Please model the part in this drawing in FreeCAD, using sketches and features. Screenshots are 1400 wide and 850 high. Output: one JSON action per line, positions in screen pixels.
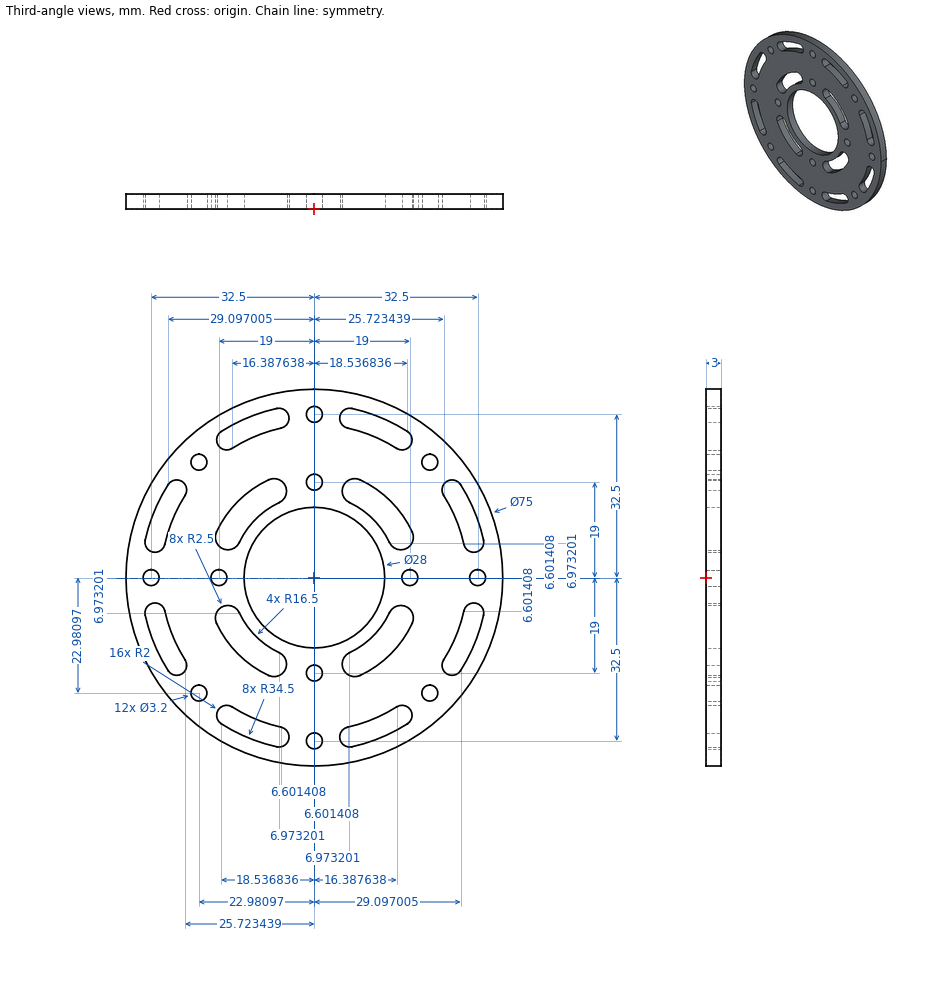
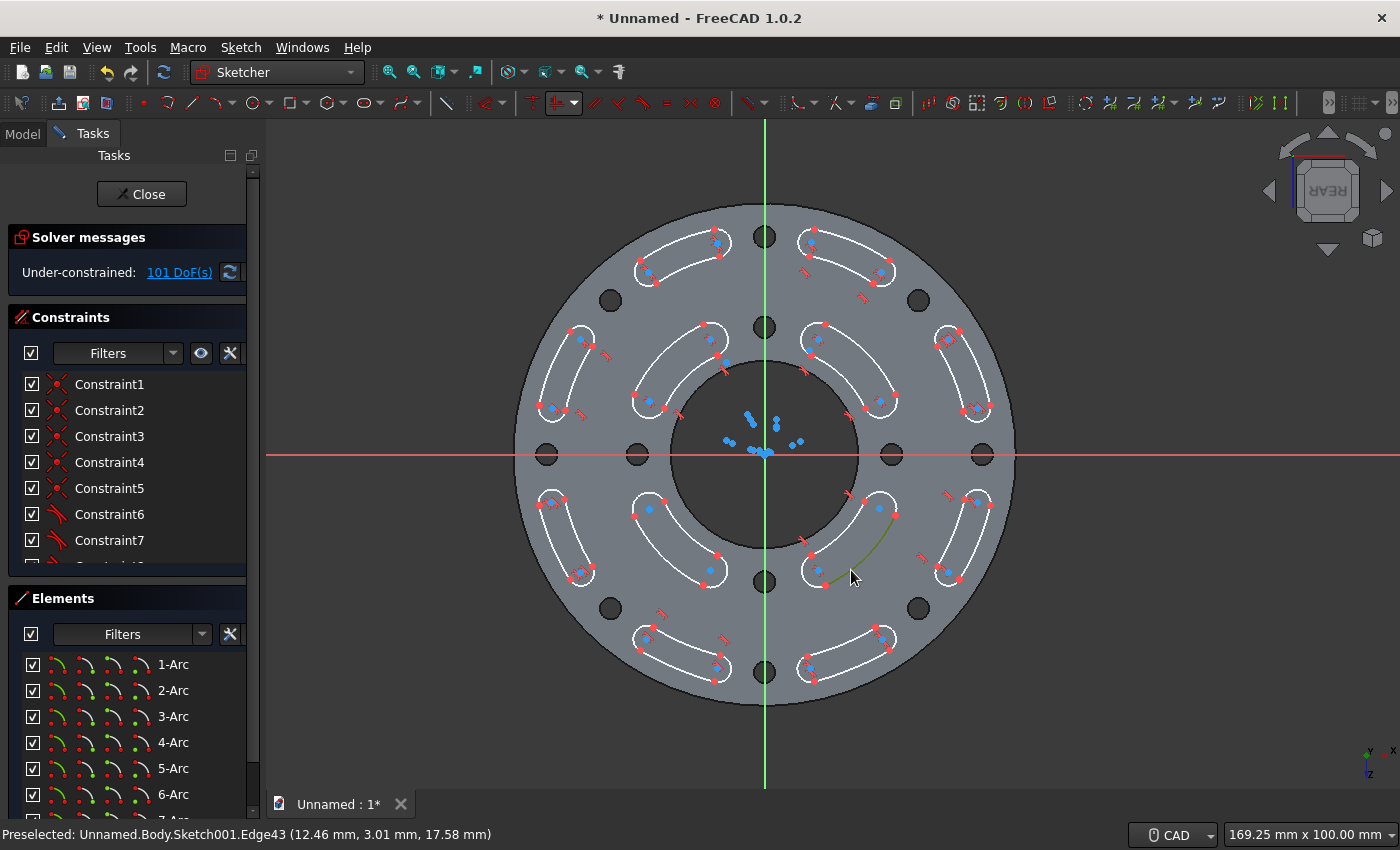
{"action": "left_click", "coordinate": [894, 501]}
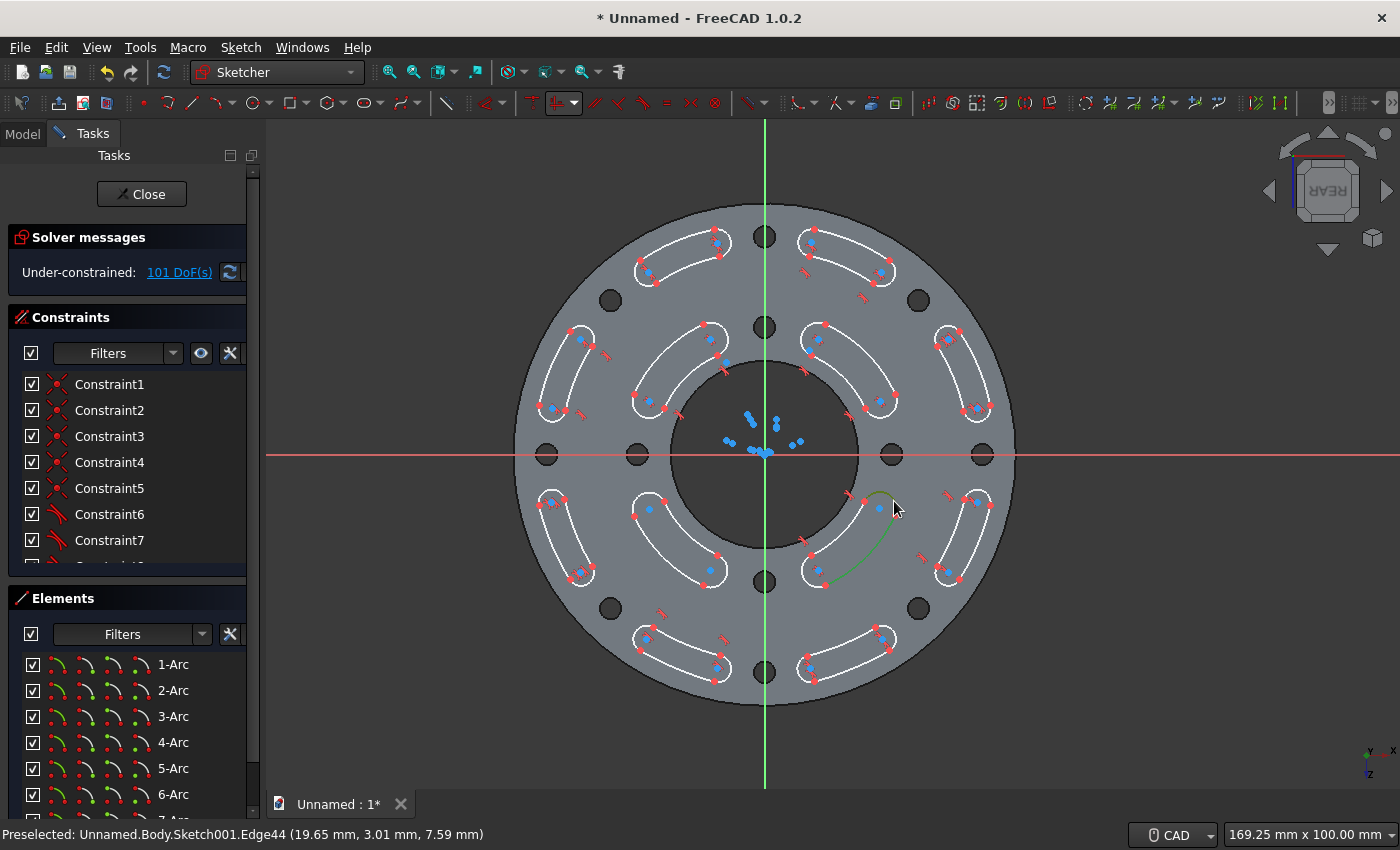
{"action": "left_click", "coordinate": [644, 104]}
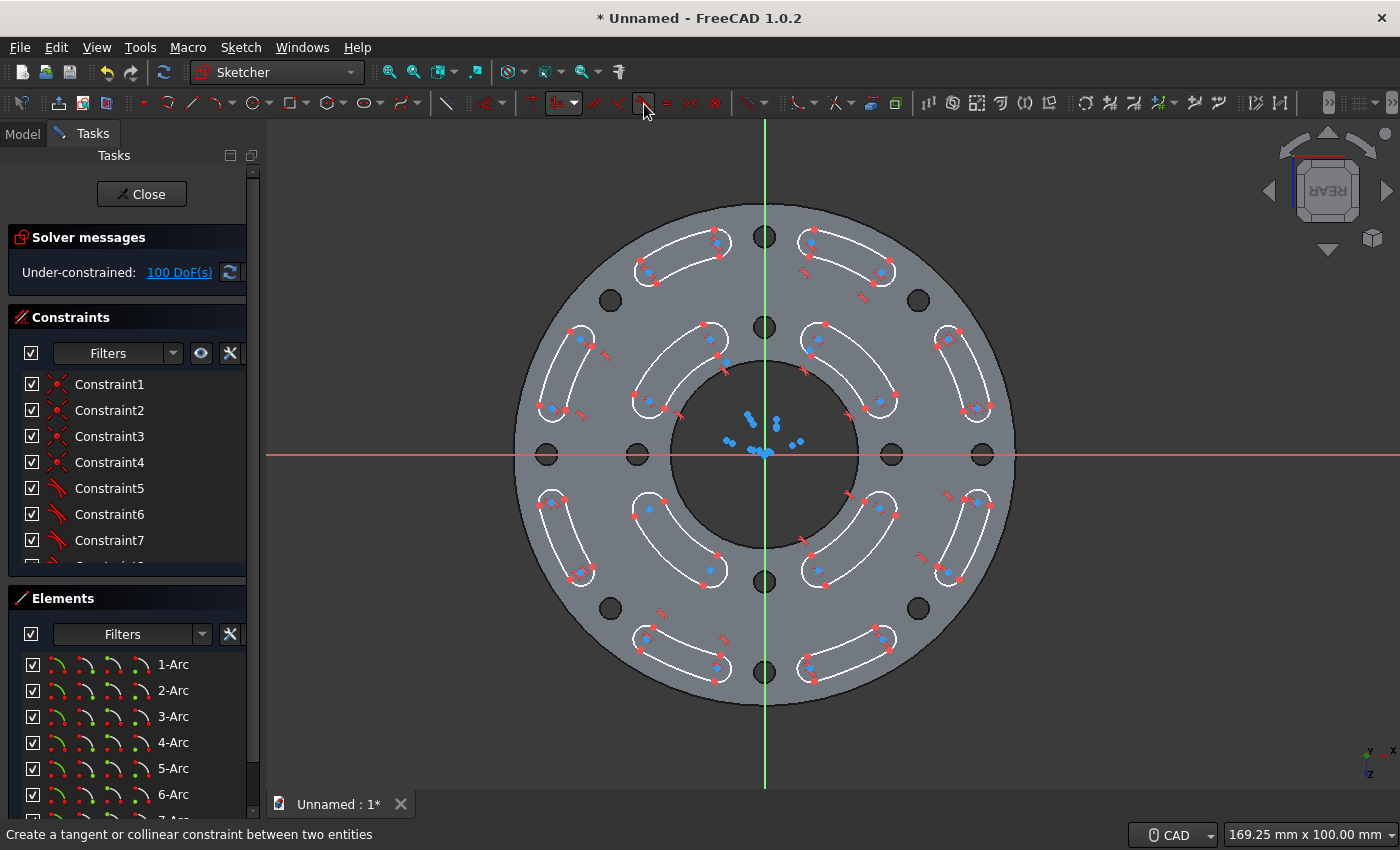
{"action": "left_click", "coordinate": [676, 521]}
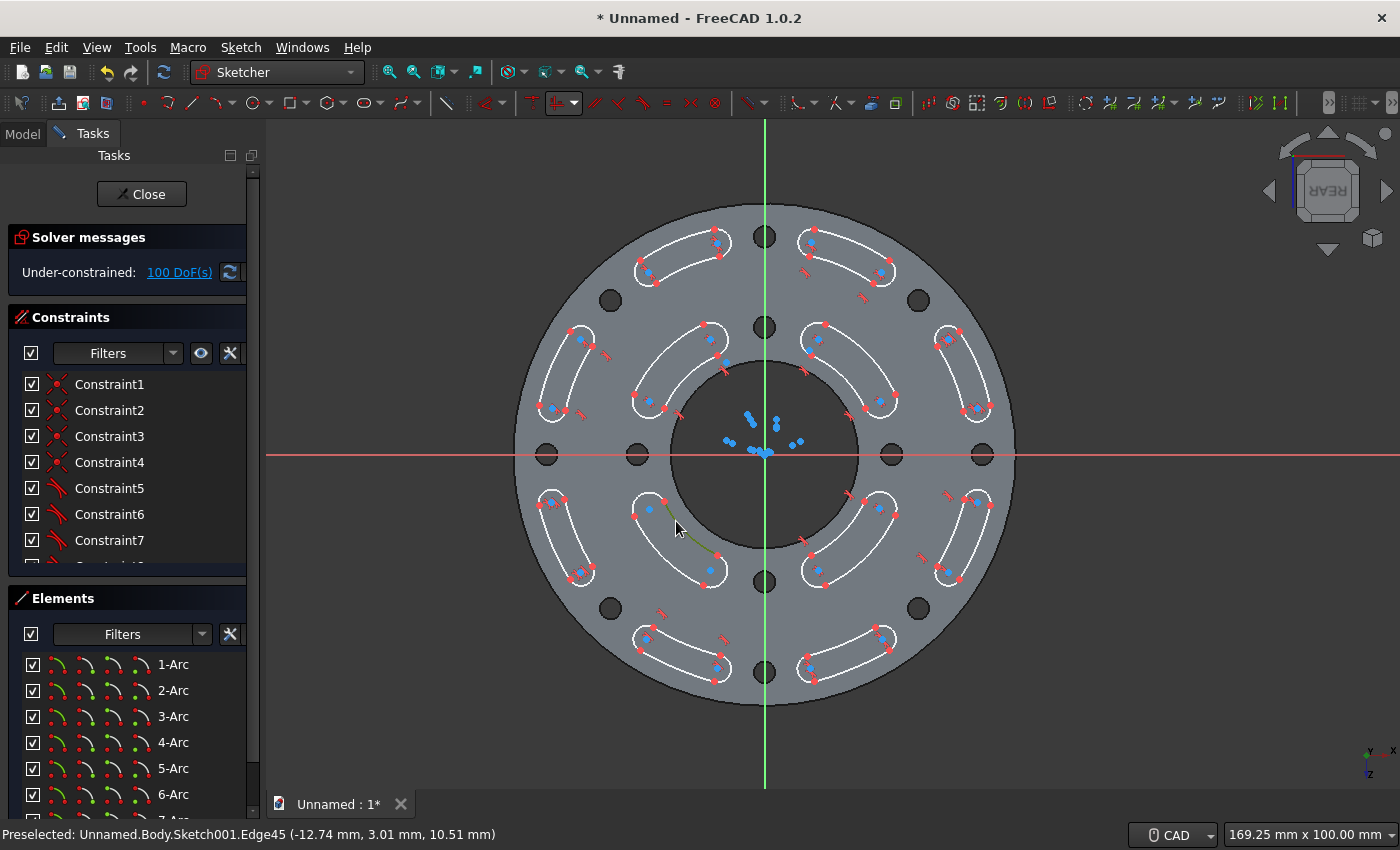
{"action": "left_click", "coordinate": [652, 493]}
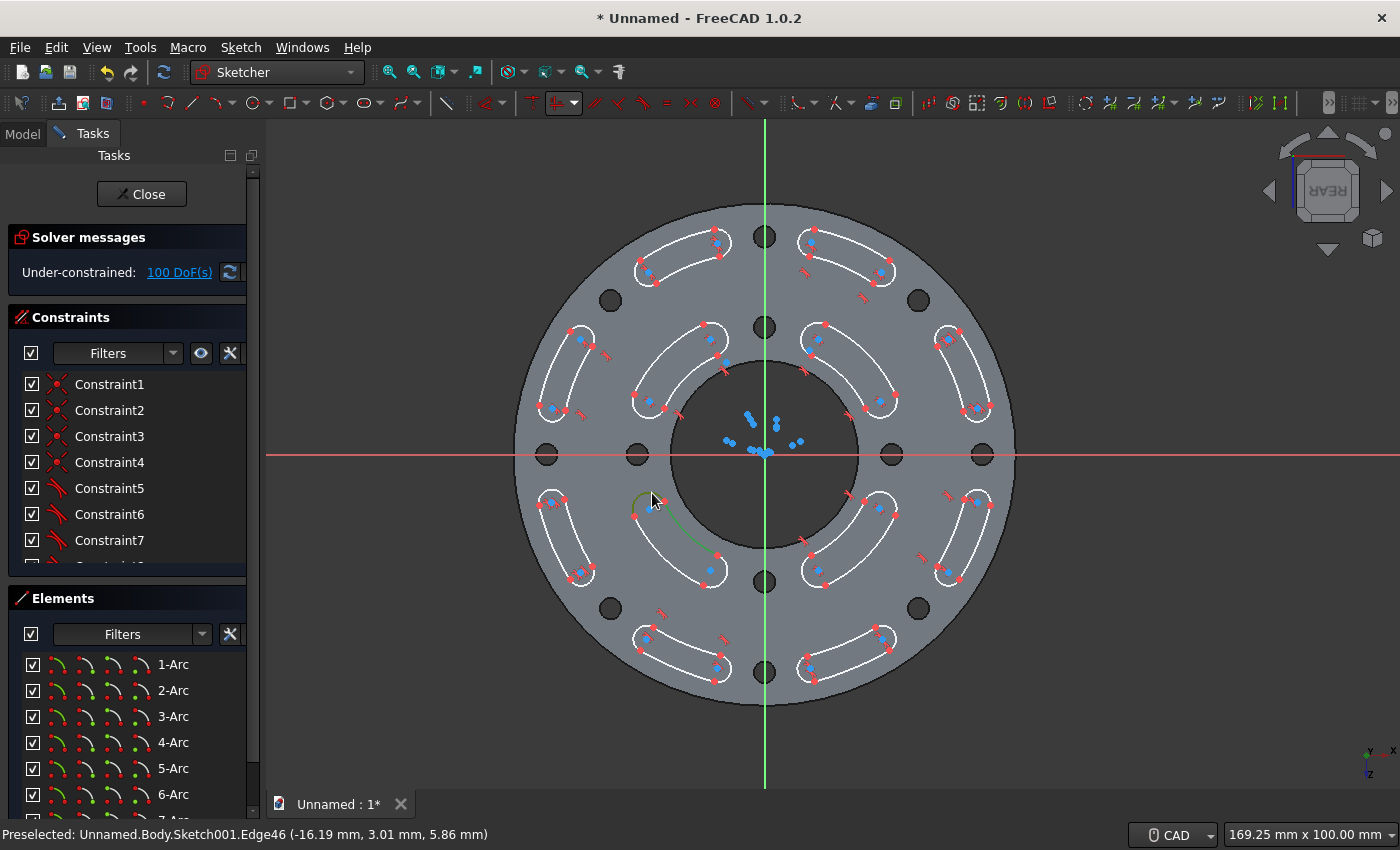
{"action": "left_click", "coordinate": [644, 104]}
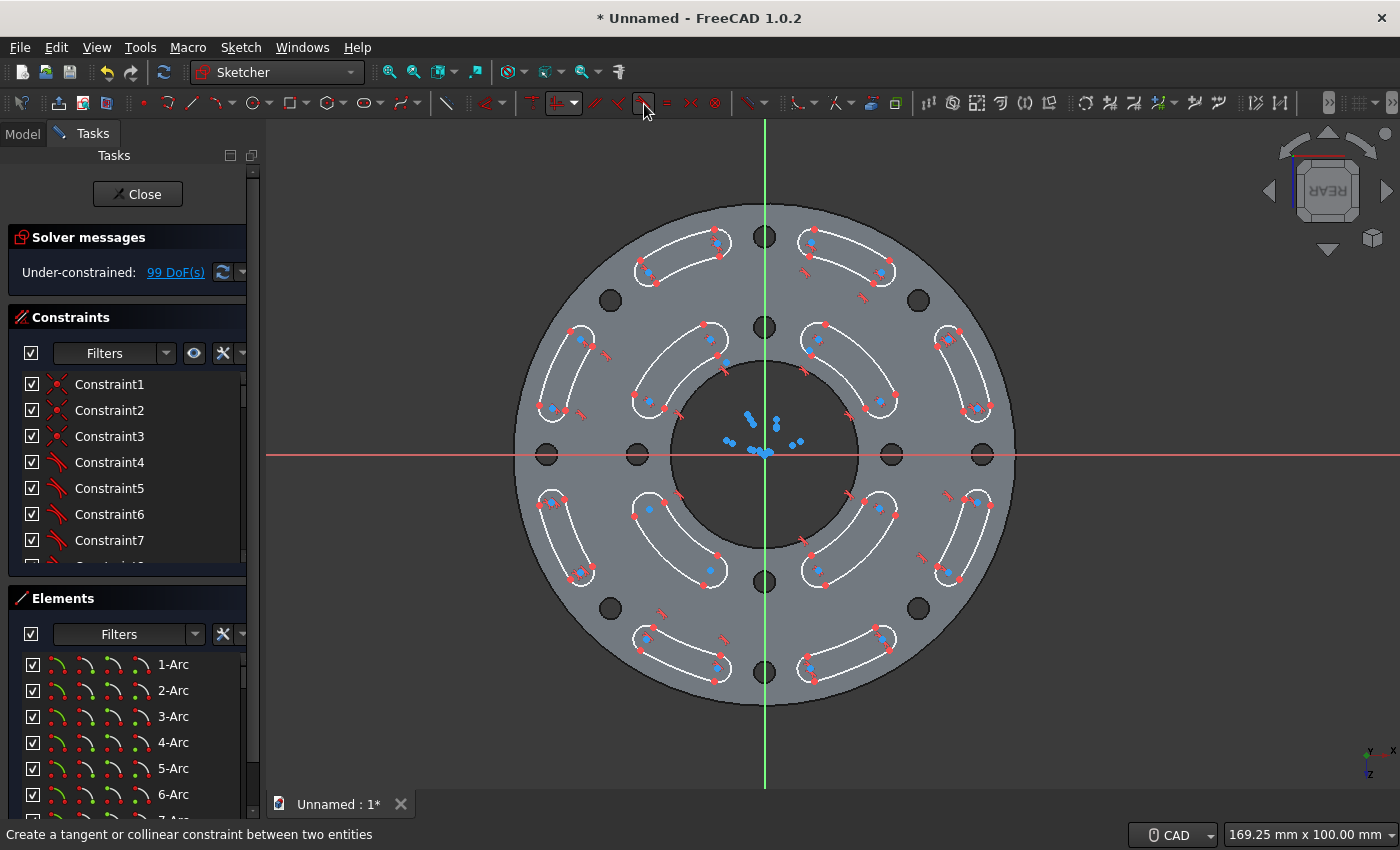
{"action": "left_click", "coordinate": [676, 522]}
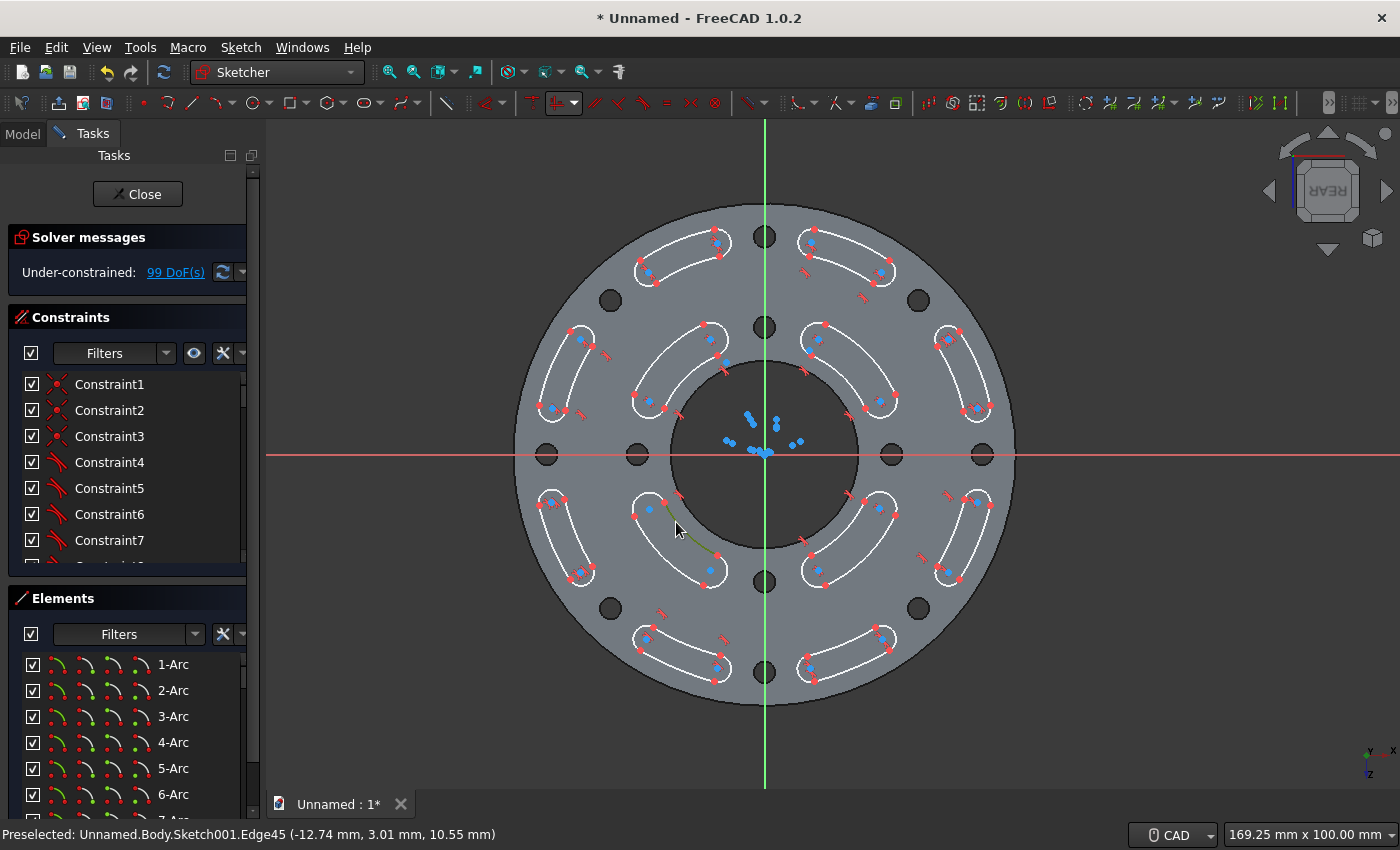
{"action": "left_click", "coordinate": [719, 585]}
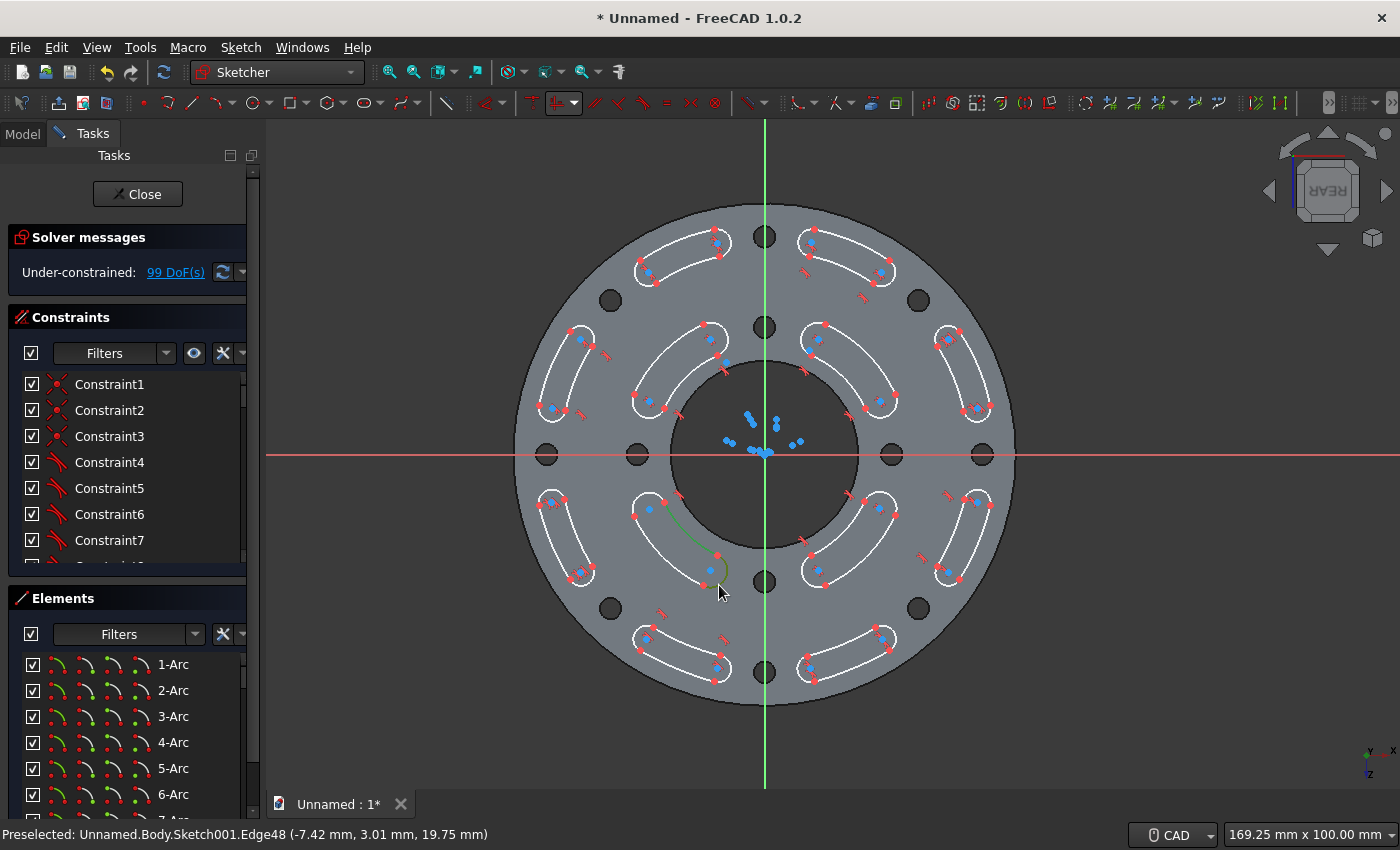
{"action": "left_click", "coordinate": [644, 104]}